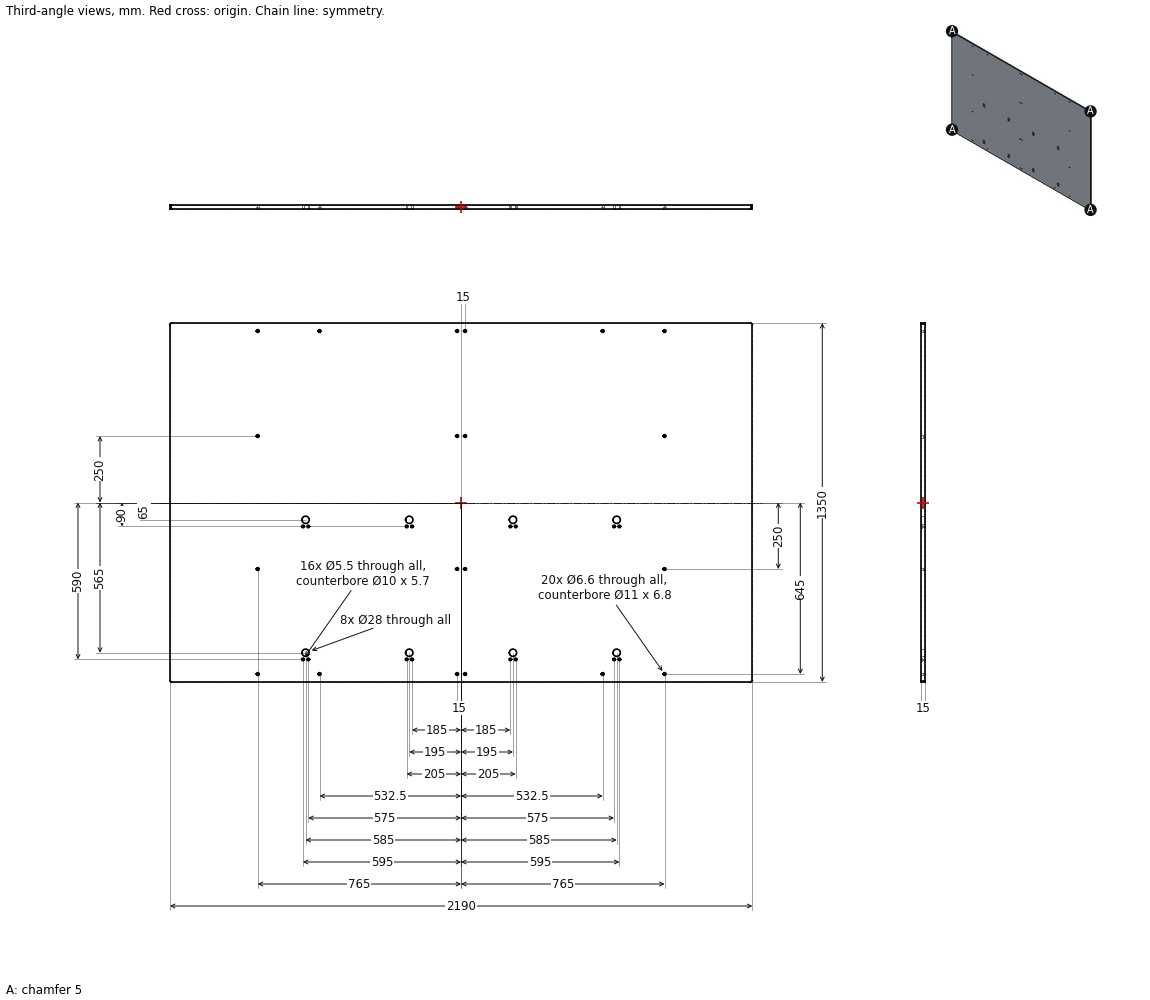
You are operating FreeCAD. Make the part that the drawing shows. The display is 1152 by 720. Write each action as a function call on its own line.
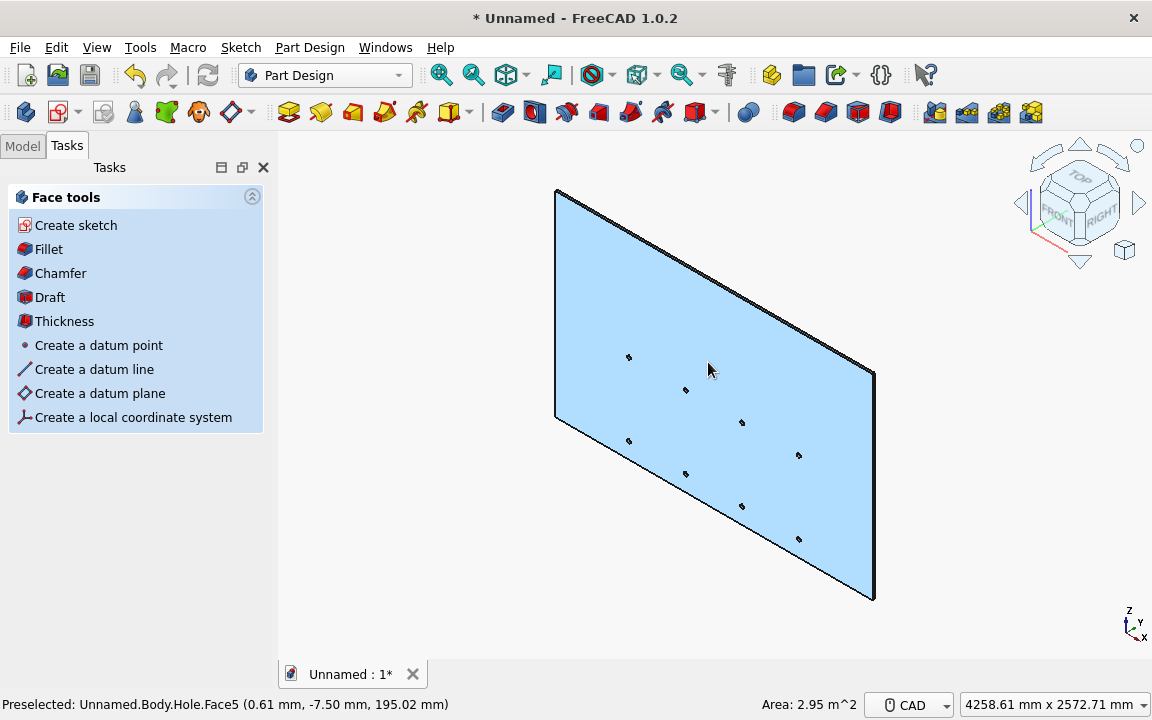
click(58, 112)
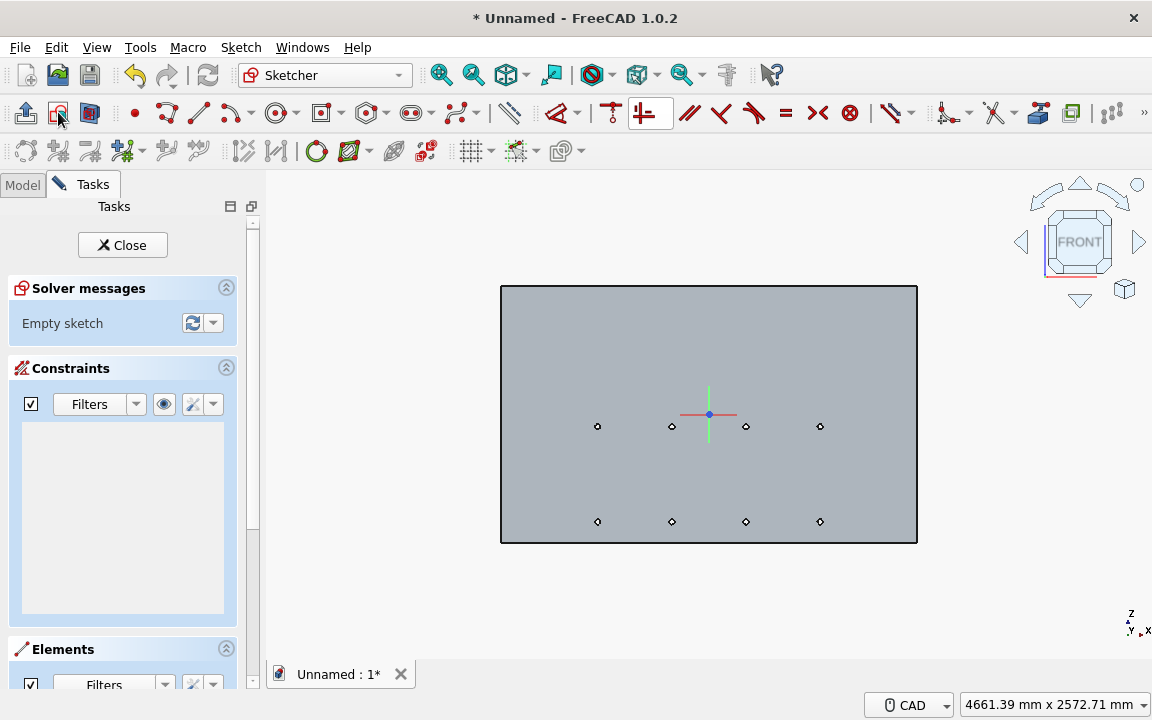
scroll(765, 517, up, 4)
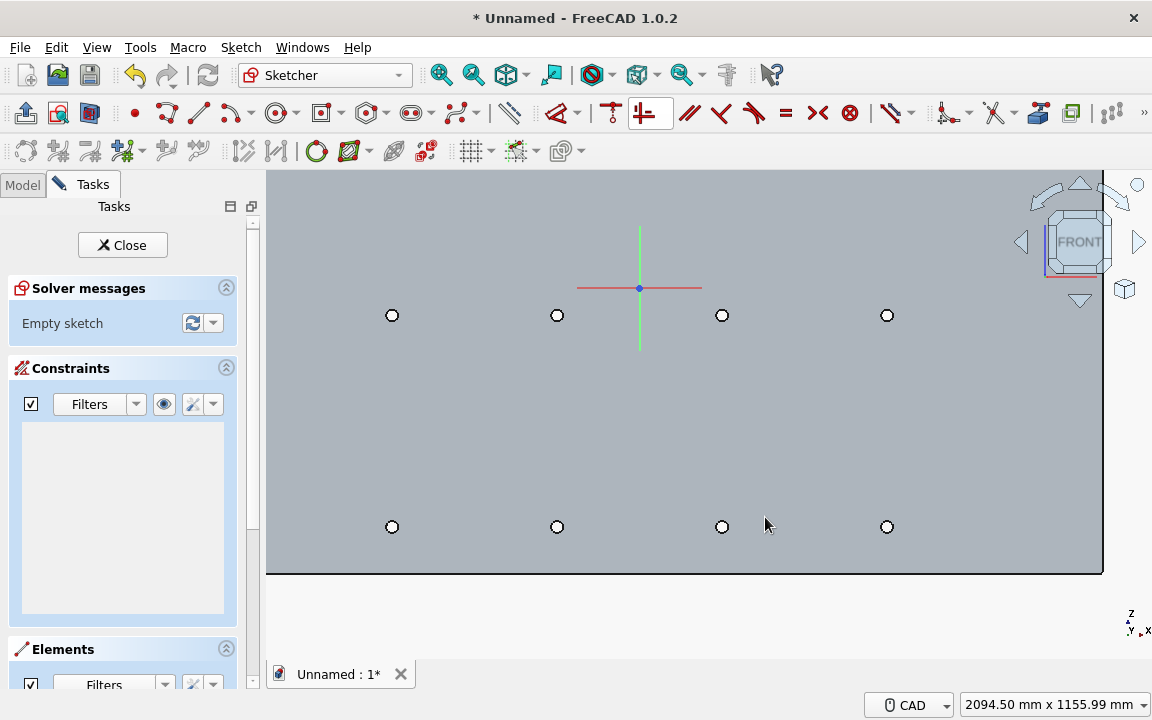
click(276, 114)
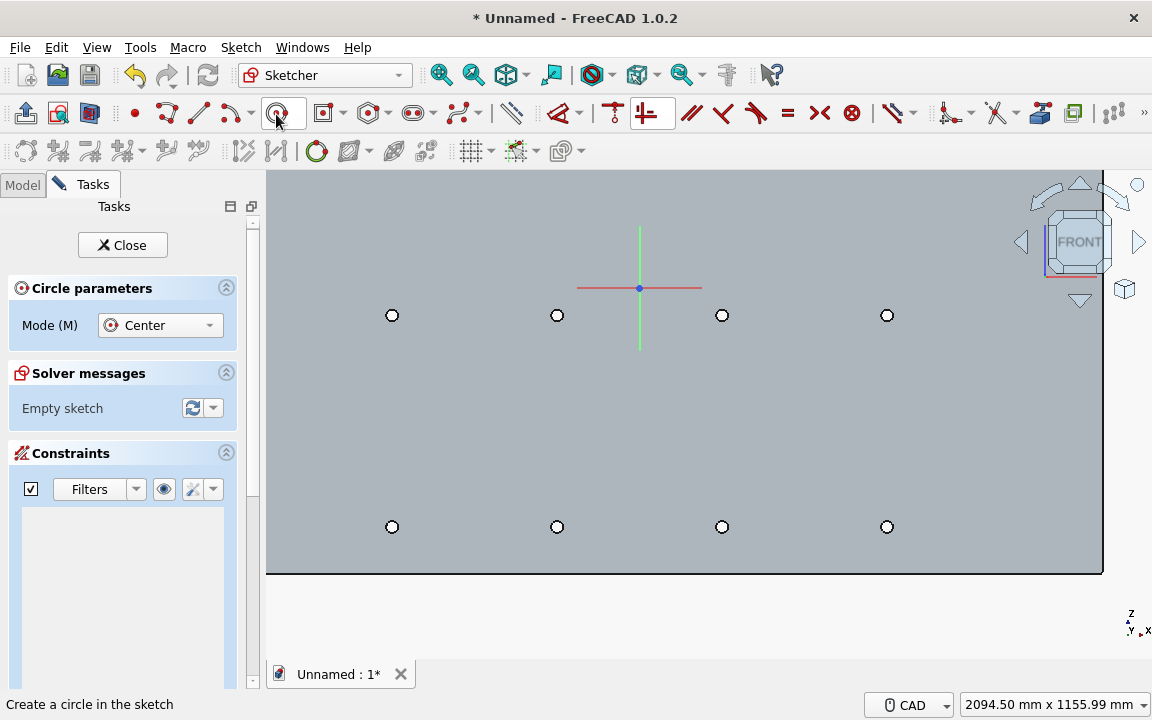
scroll(388, 538, up, 15)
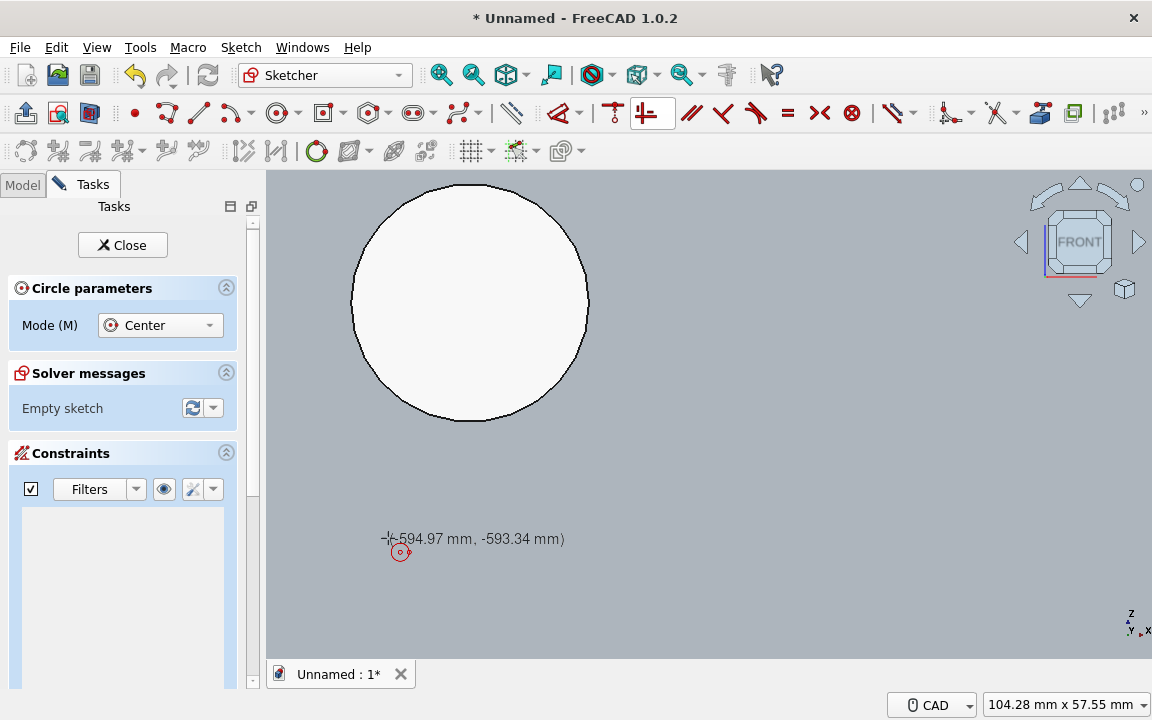
scroll(389, 540, down, 15)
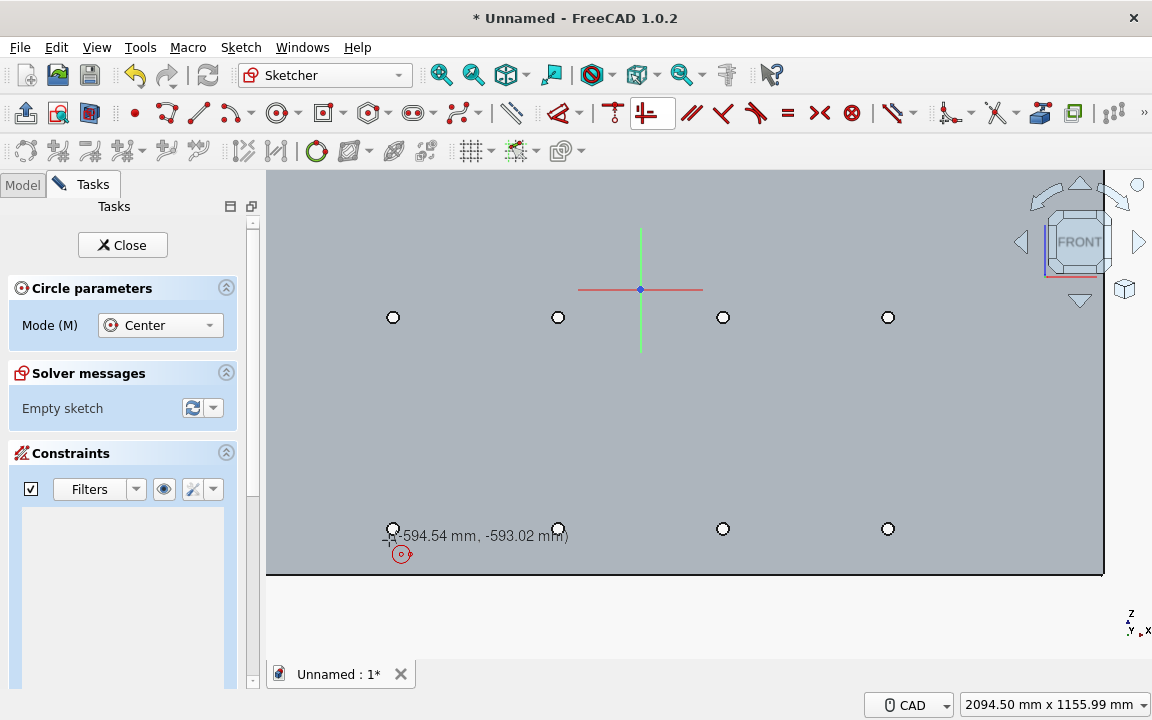
click(389, 539)
move(390, 539)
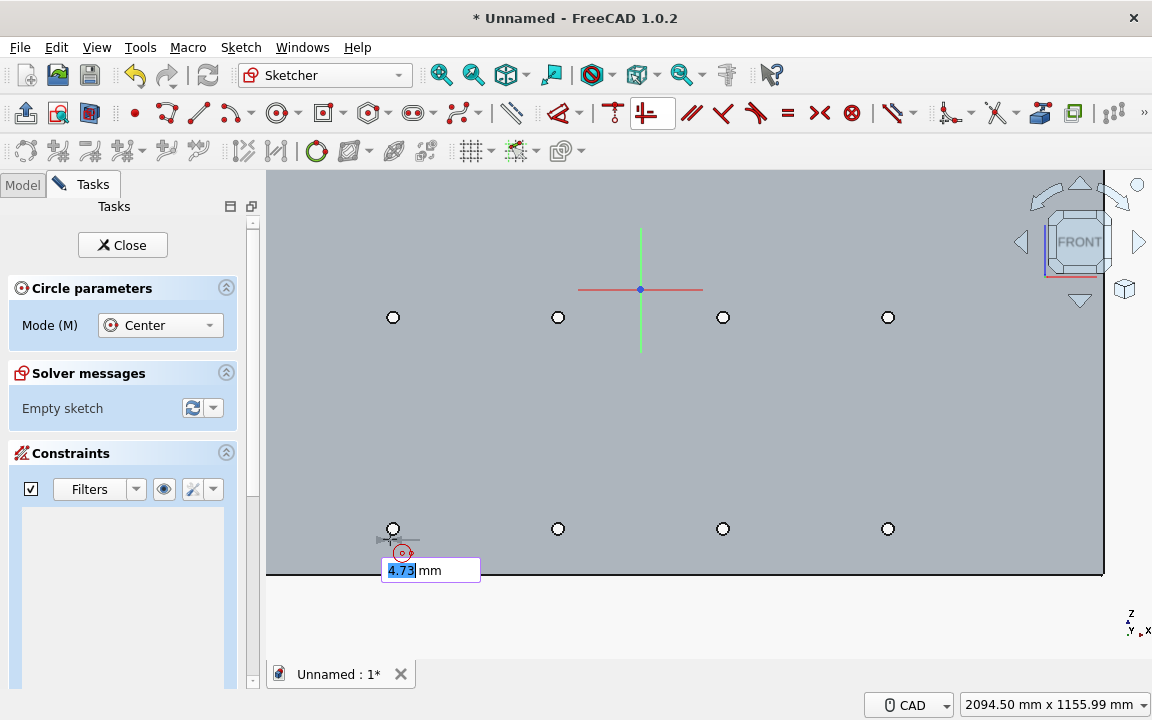
text(5.5)
key(Return)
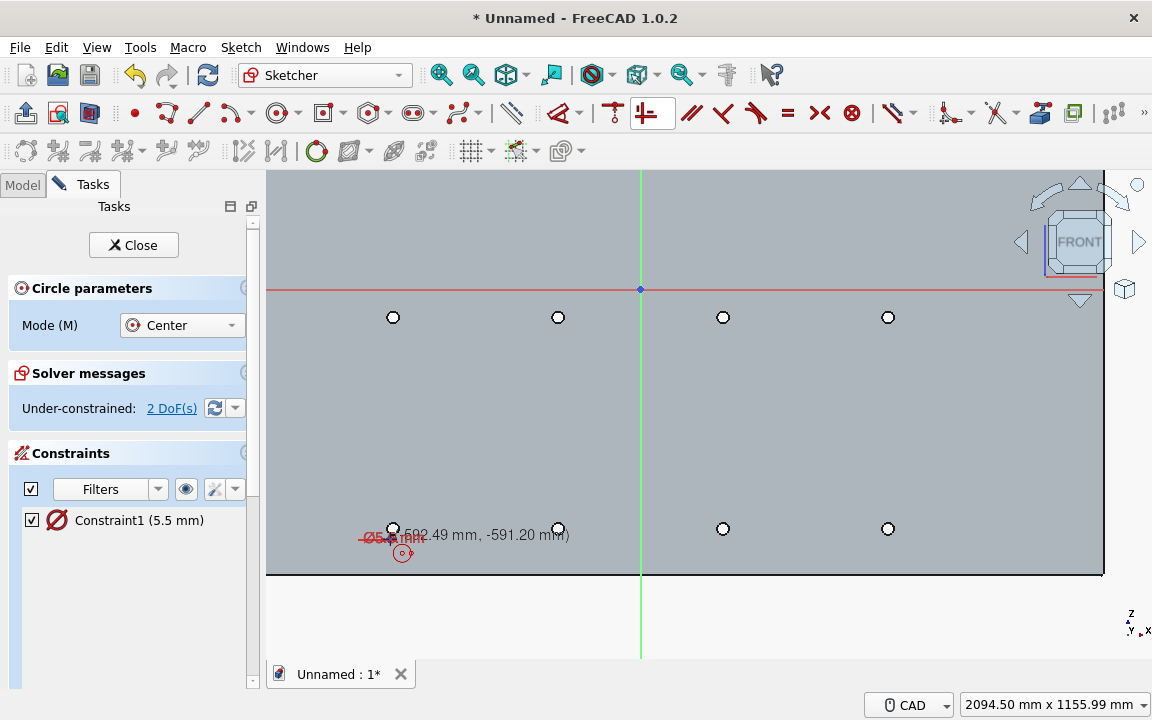
scroll(397, 539, up, 15)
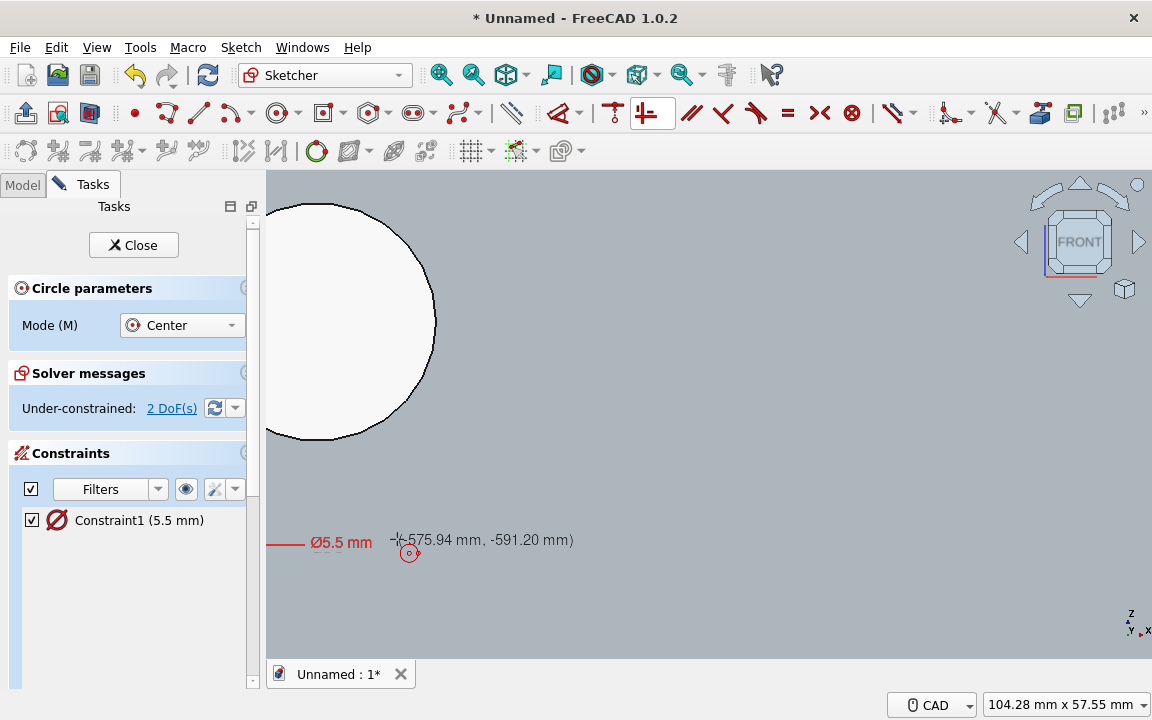
scroll(397, 539, down, 15)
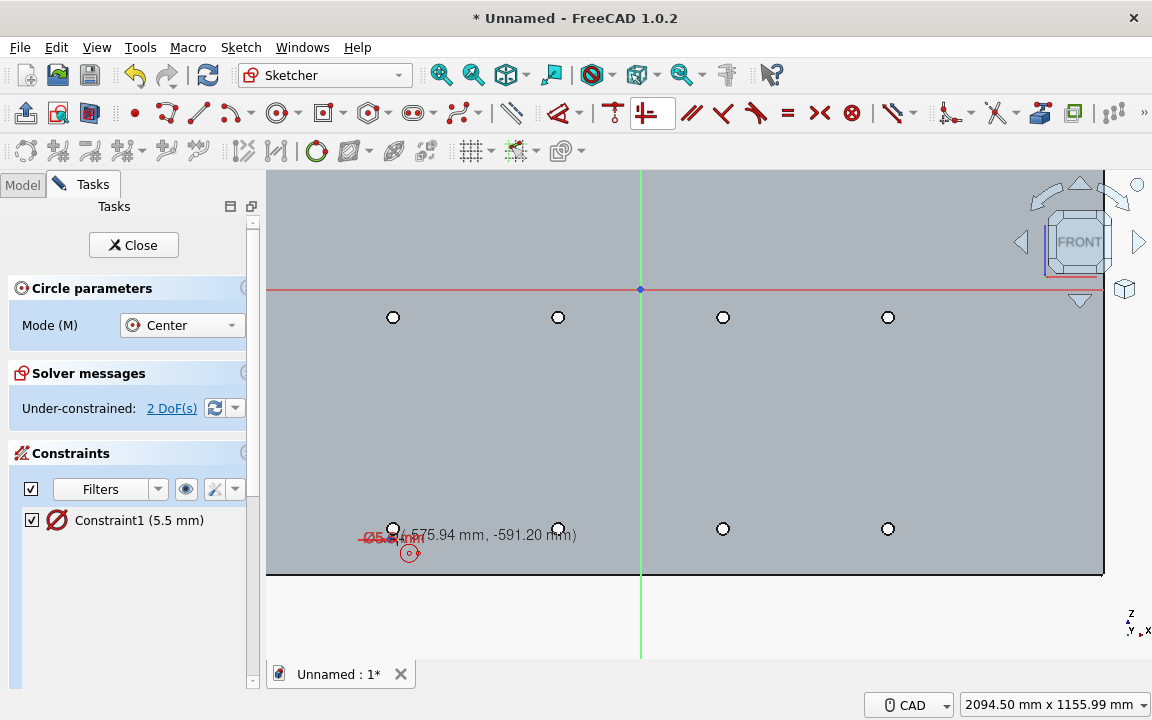
scroll(397, 539, up, 4)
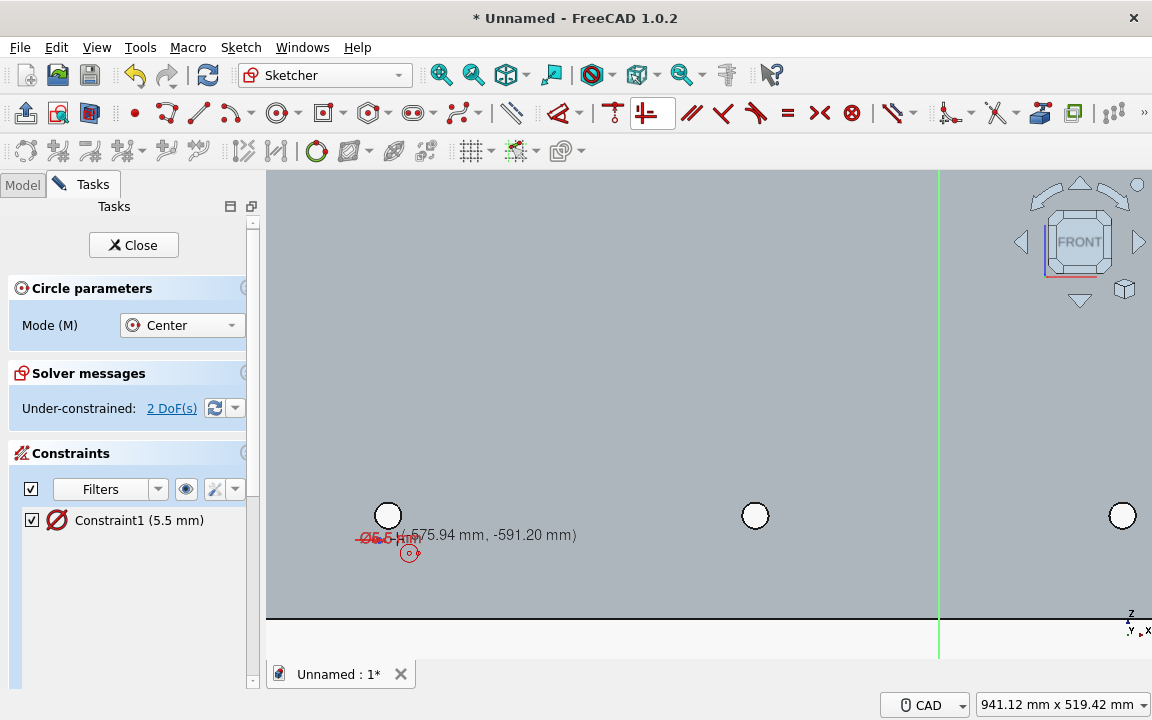
click(398, 539)
move(400, 537)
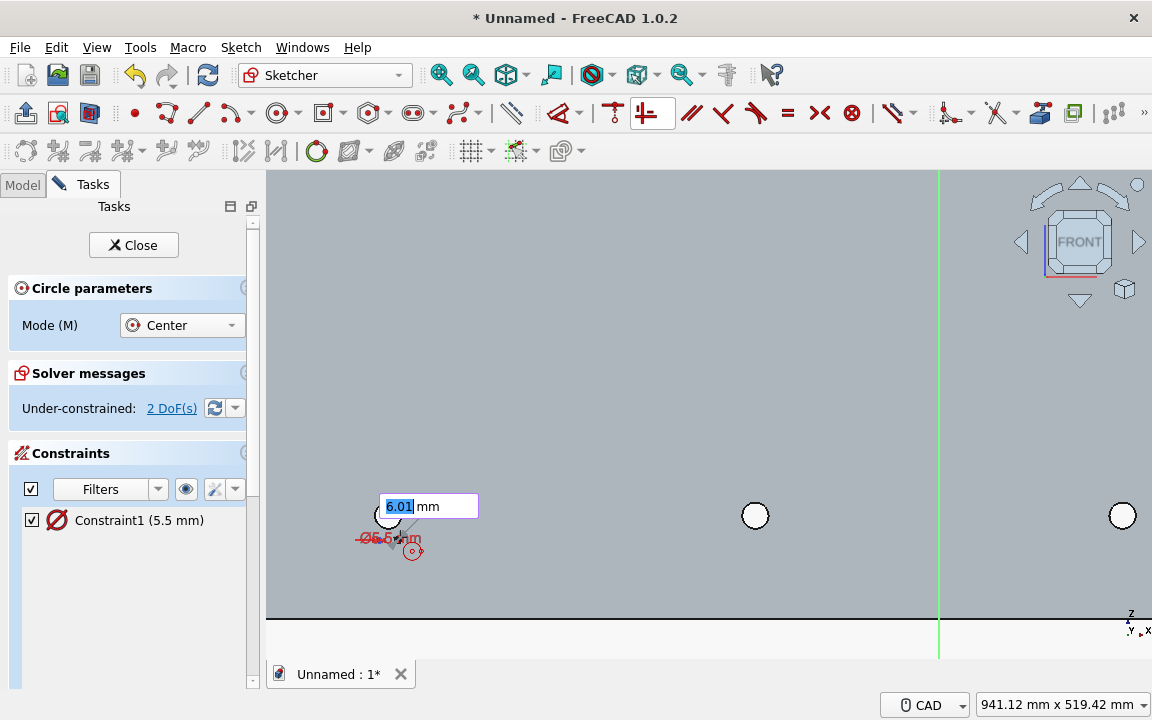
text(5.5)
key(Return)